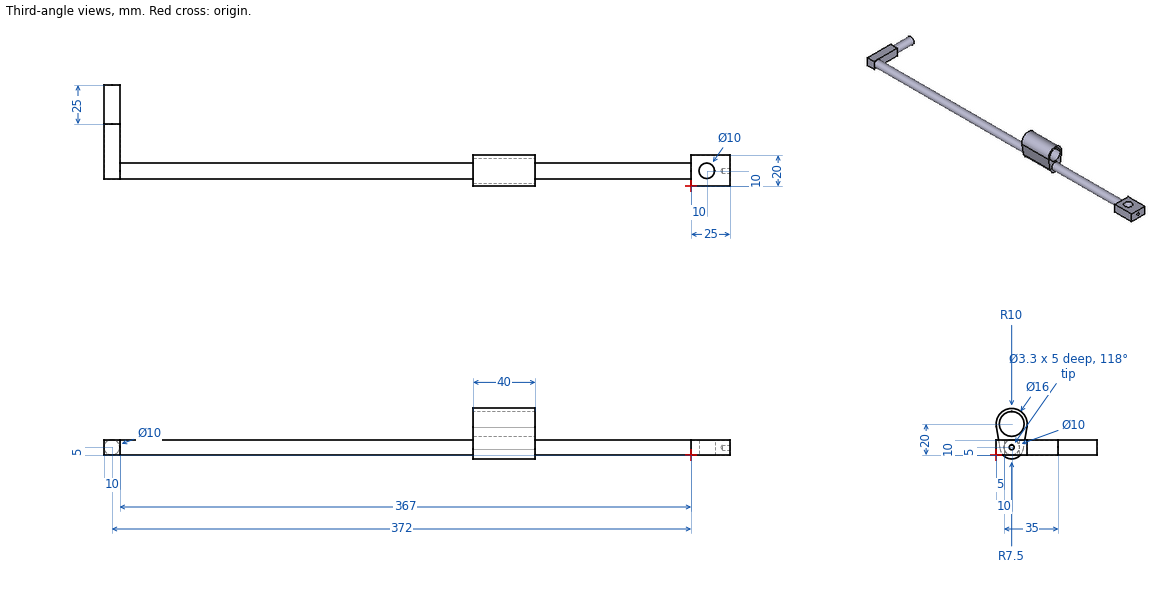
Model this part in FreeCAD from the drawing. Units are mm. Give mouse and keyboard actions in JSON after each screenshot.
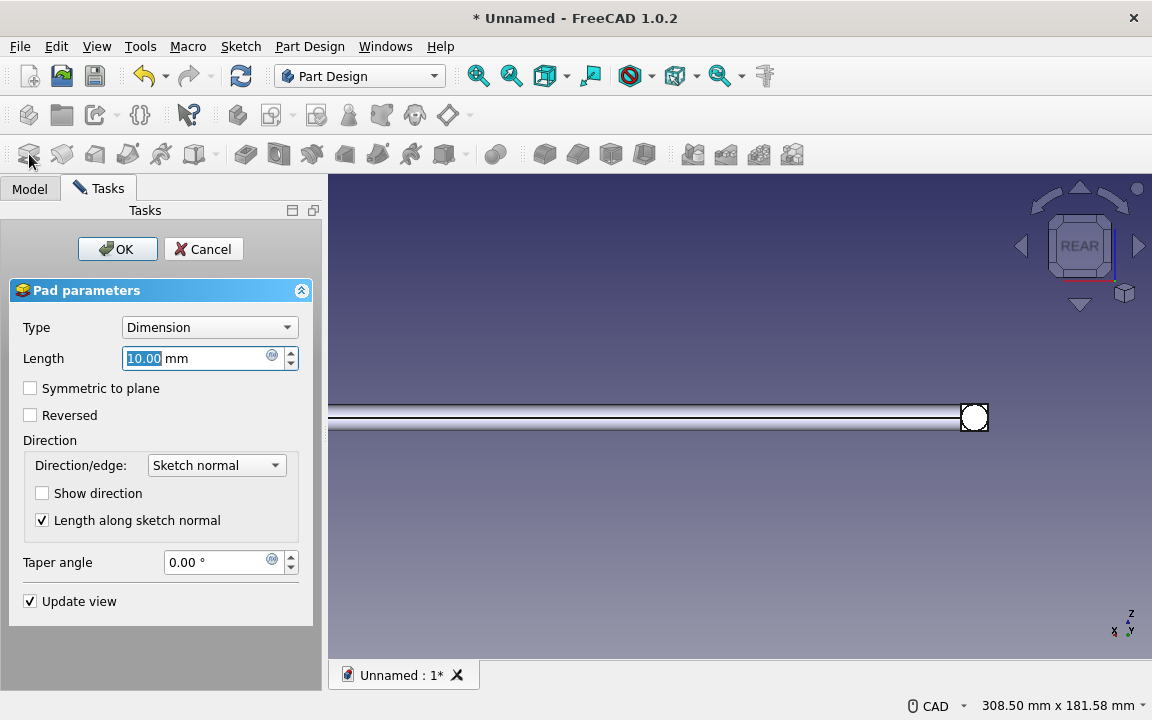
{"action": "type", "text": "25"}
{"action": "key", "text": "Tab"}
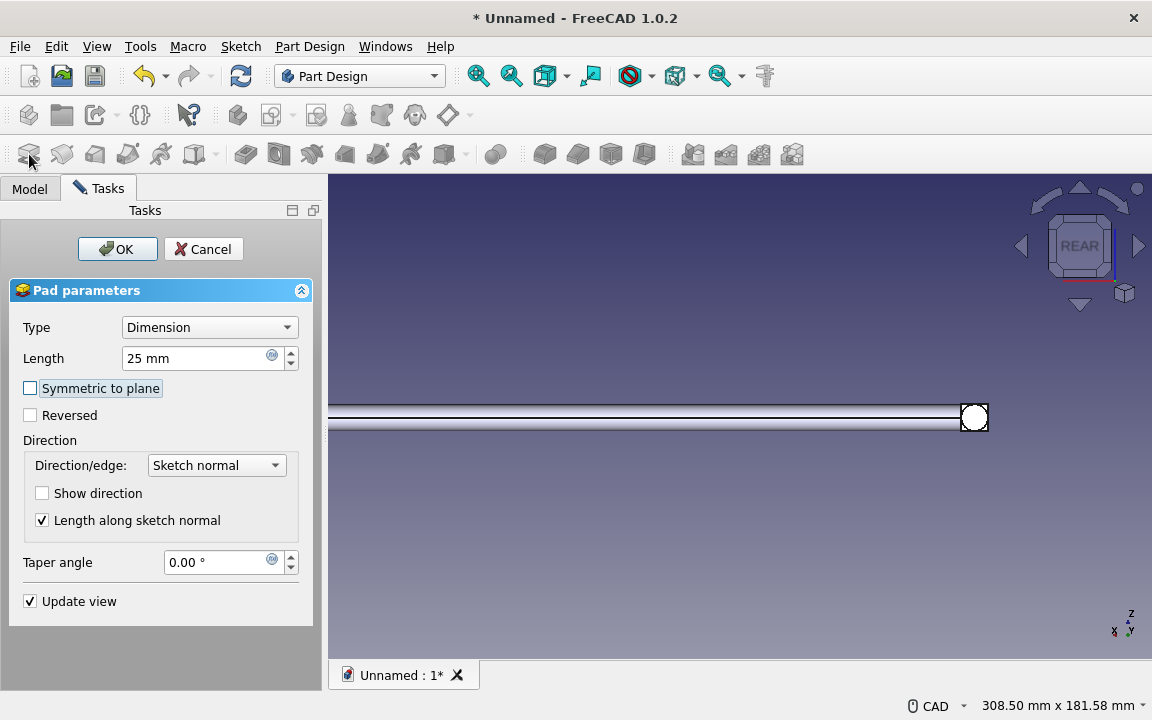
{"action": "left_click", "coordinate": [118, 249]}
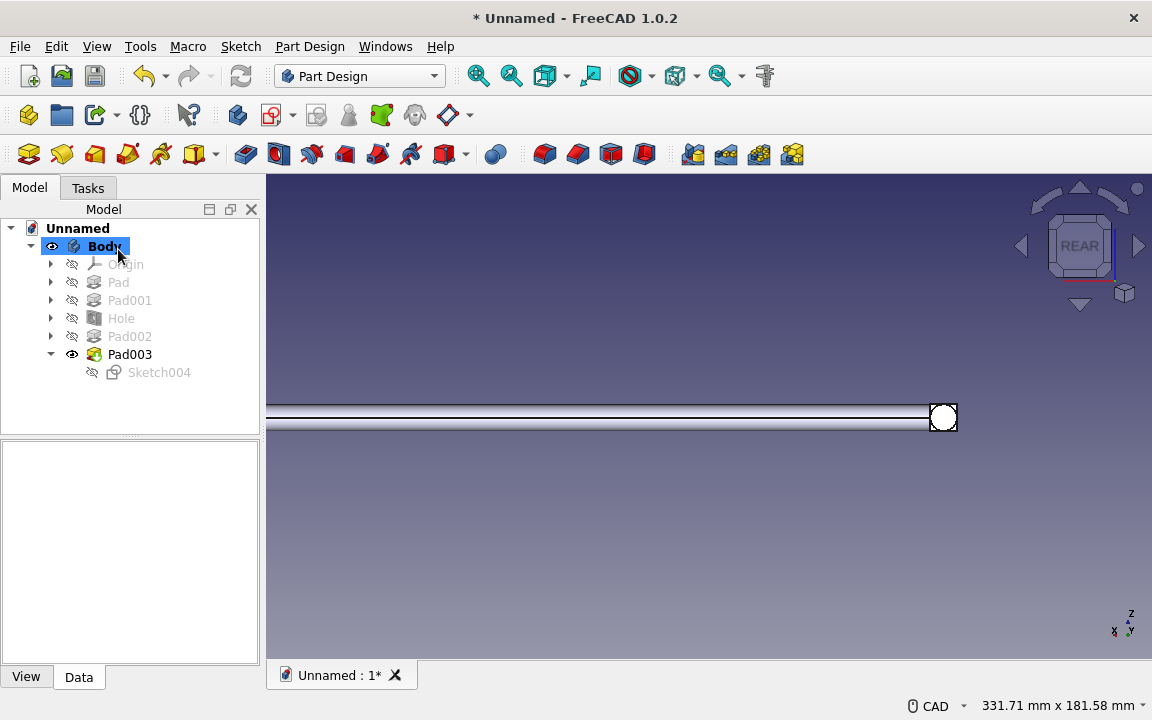
{"action": "key", "text": "v f"}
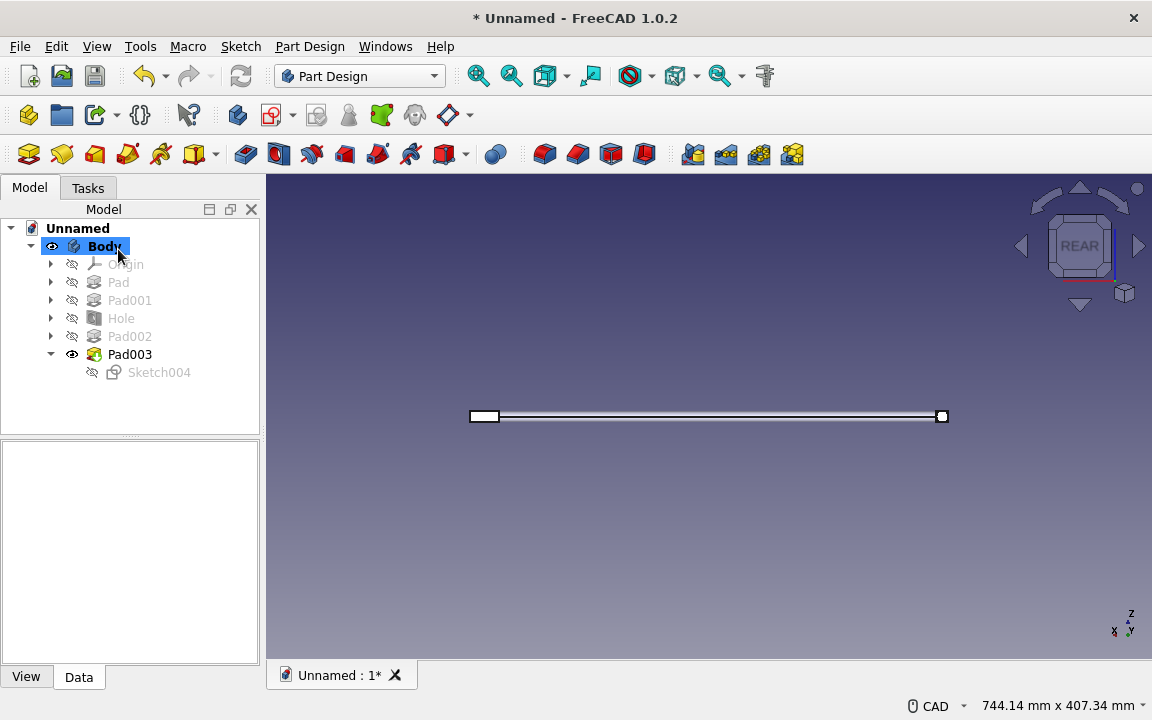
{"action": "left_click", "coordinate": [51, 264]}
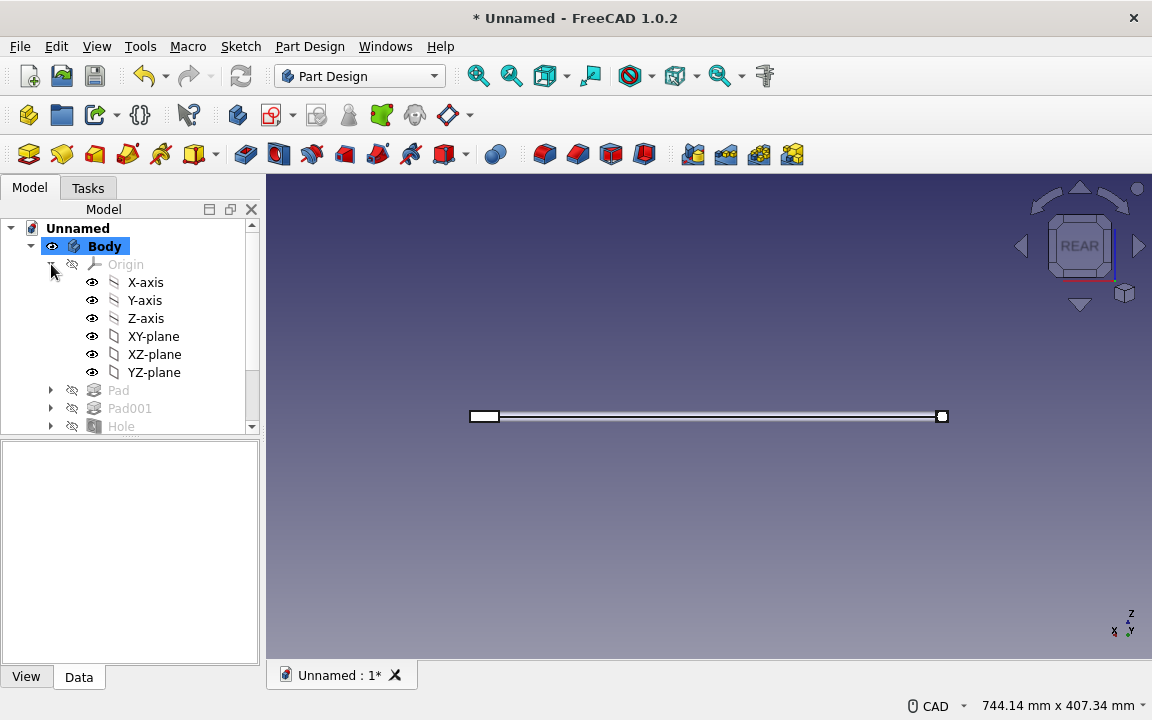
{"action": "left_click", "coordinate": [137, 372]}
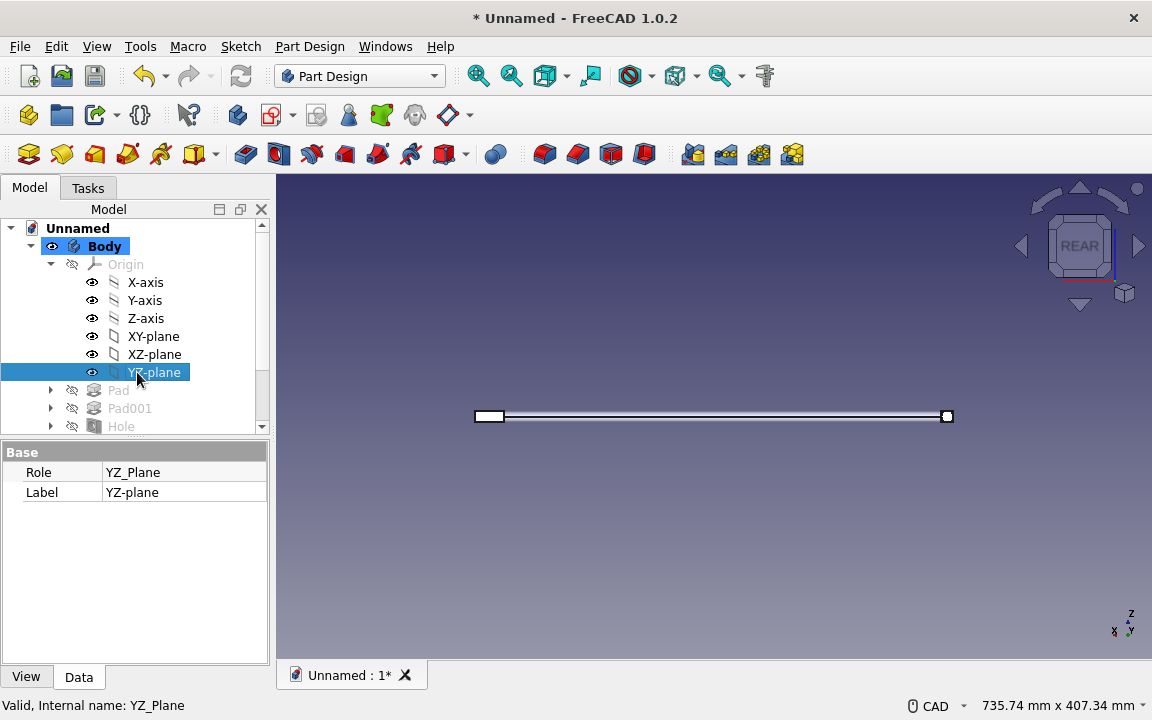
{"action": "left_click", "coordinate": [448, 116]}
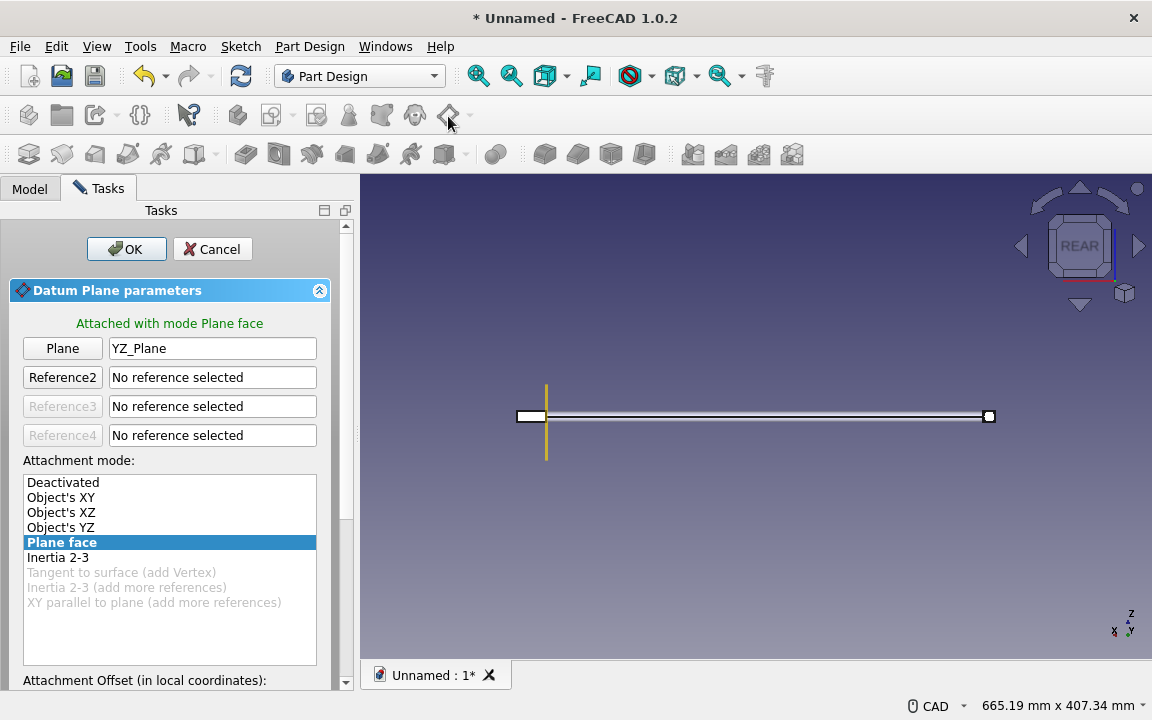
{"action": "scroll", "coordinate": [346, 455], "scroll_direction": "down", "scroll_amount": 3}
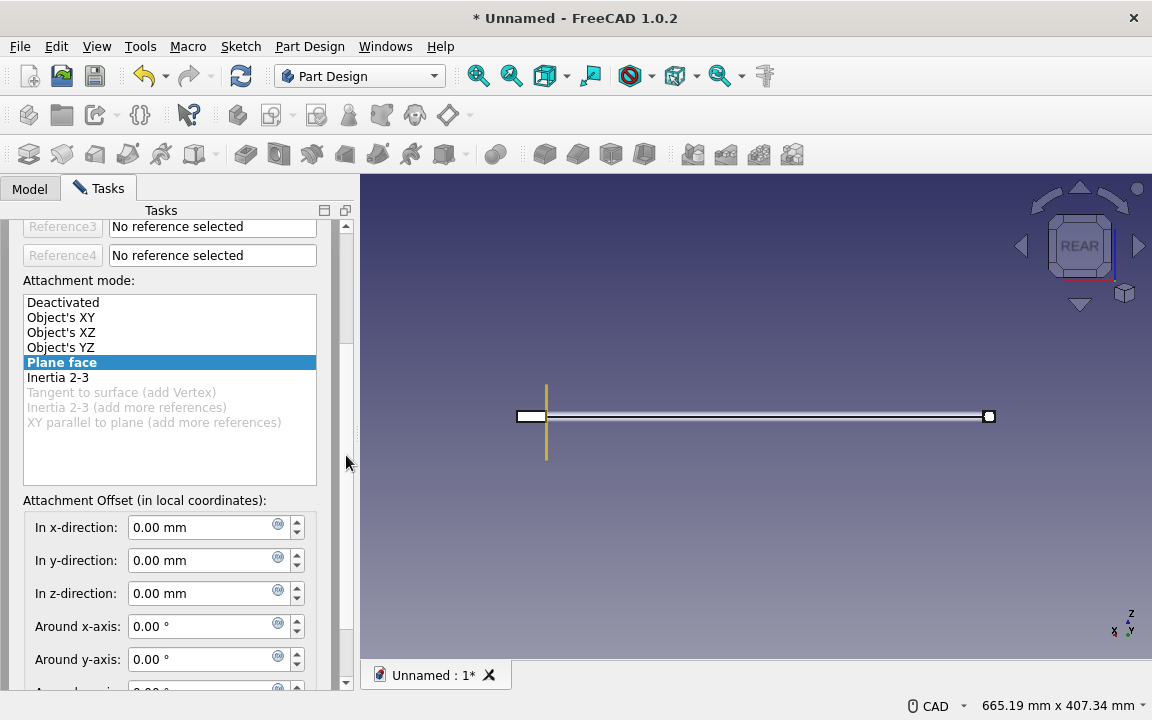
{"action": "triple_click", "coordinate": [210, 594]}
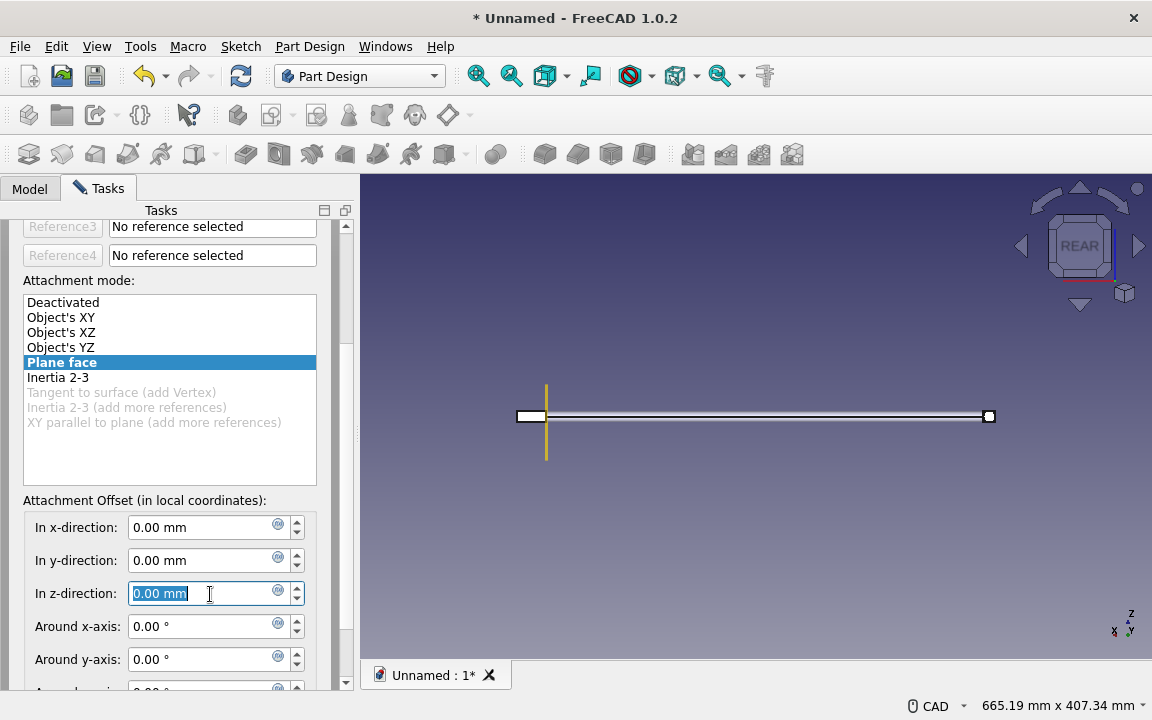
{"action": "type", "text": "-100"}
{"action": "key", "text": "Tab"}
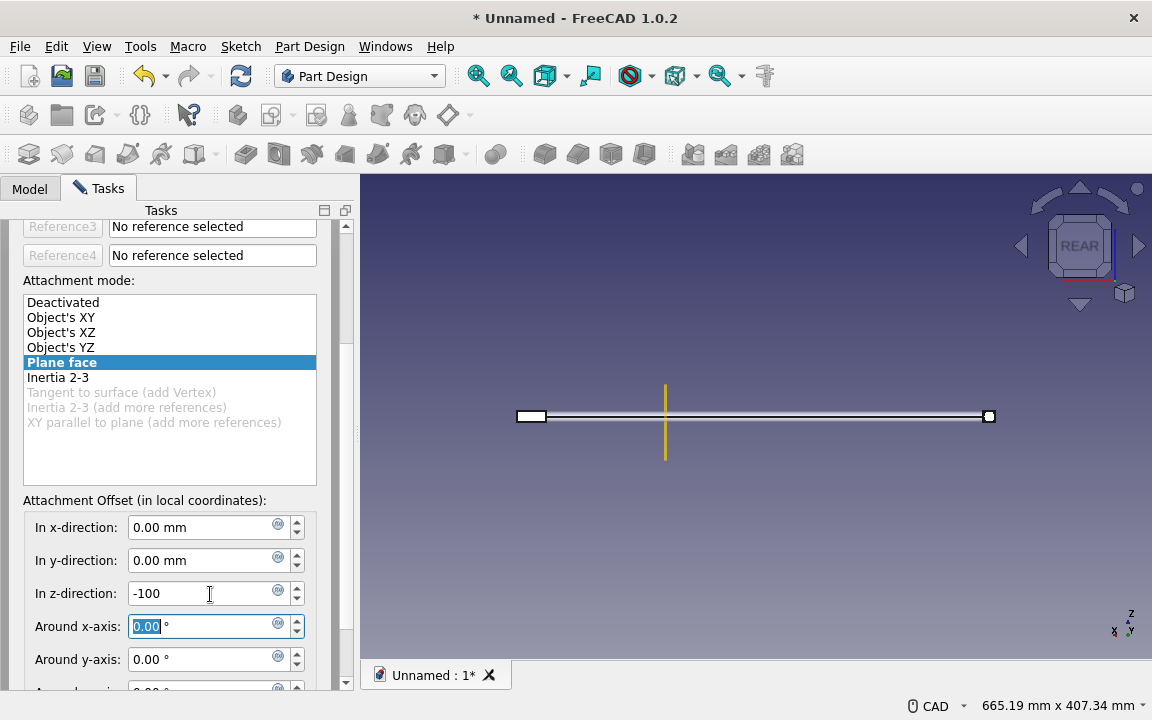
{"action": "scroll", "coordinate": [346, 455], "scroll_direction": "up", "scroll_amount": 4}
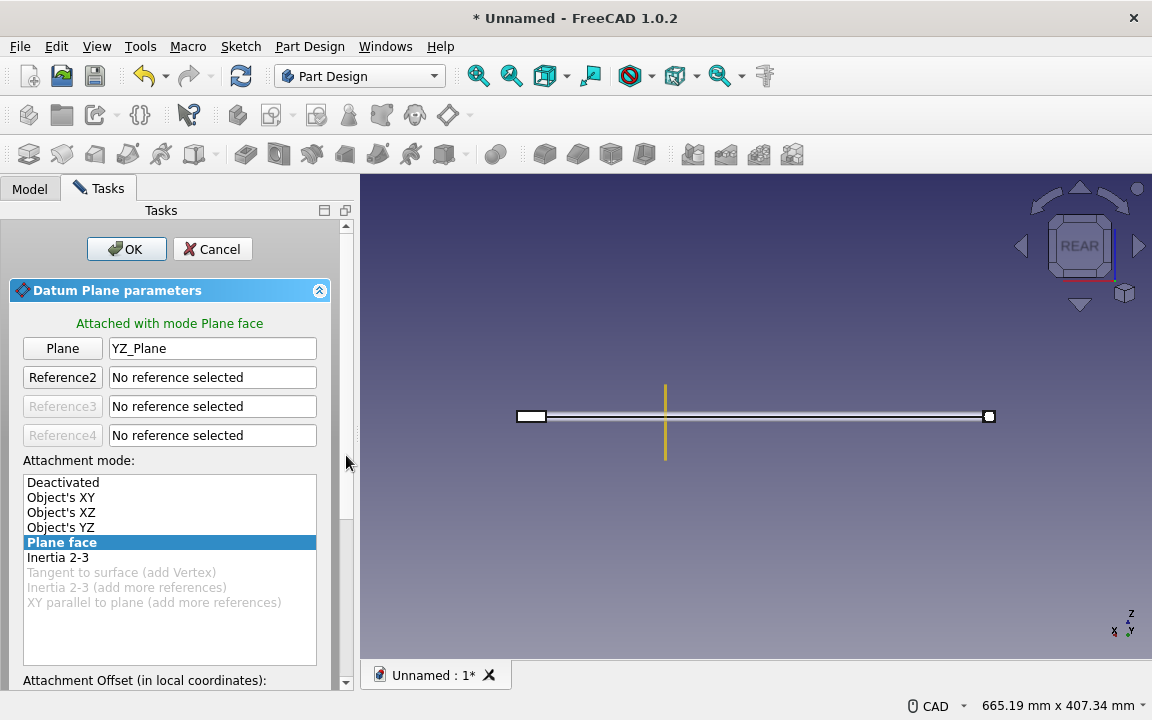
{"action": "left_click", "coordinate": [127, 249]}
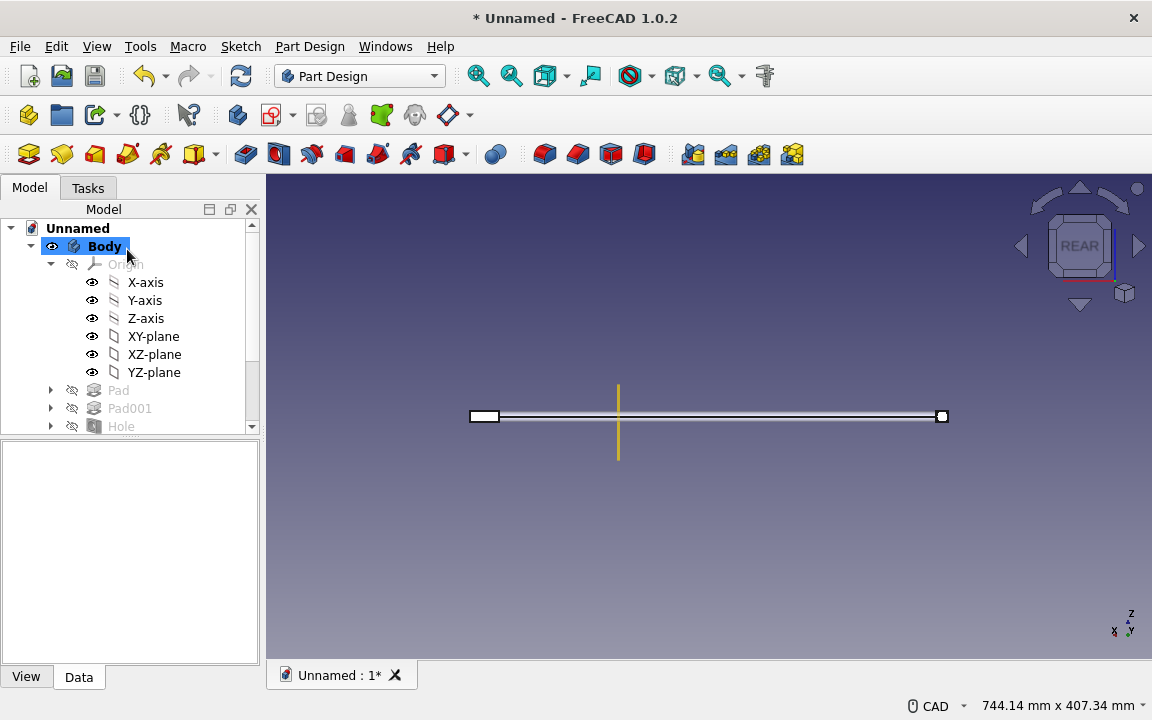
{"action": "scroll", "coordinate": [101, 332], "scroll_direction": "down", "scroll_amount": 3}